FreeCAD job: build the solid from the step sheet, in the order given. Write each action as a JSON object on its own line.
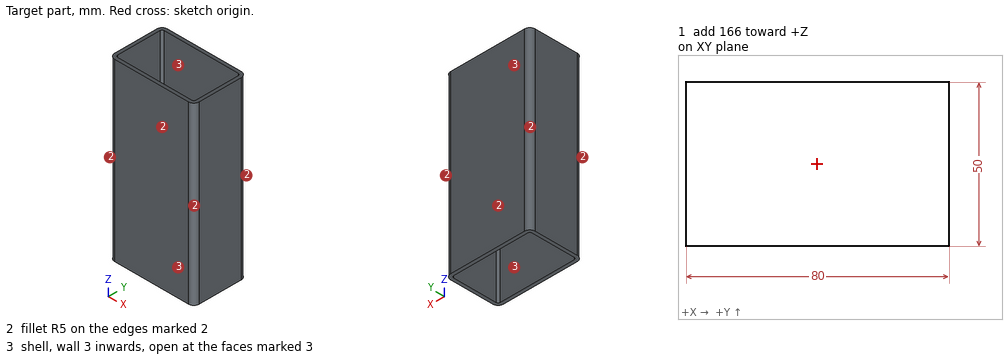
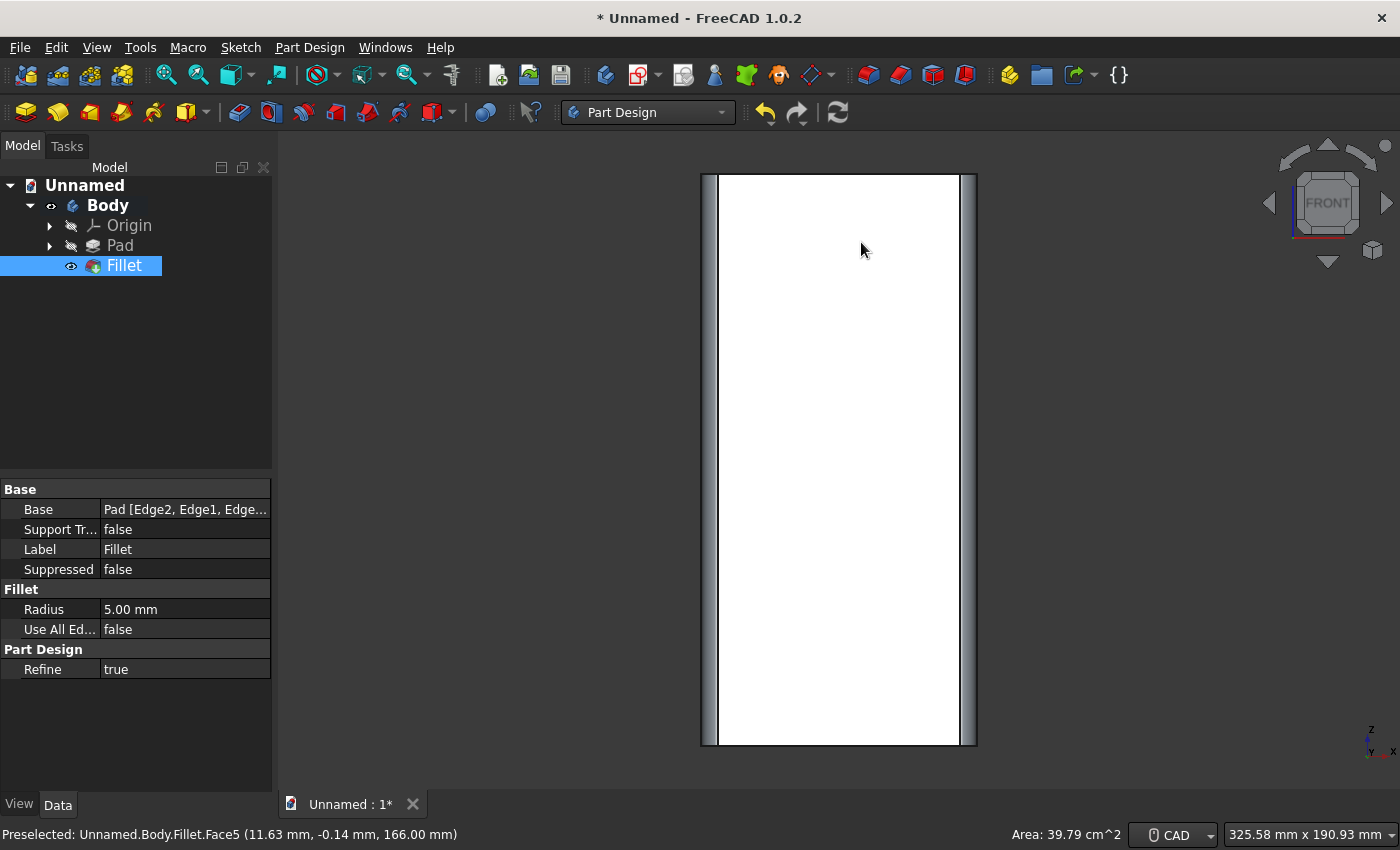
{"action": "key", "text": "3"}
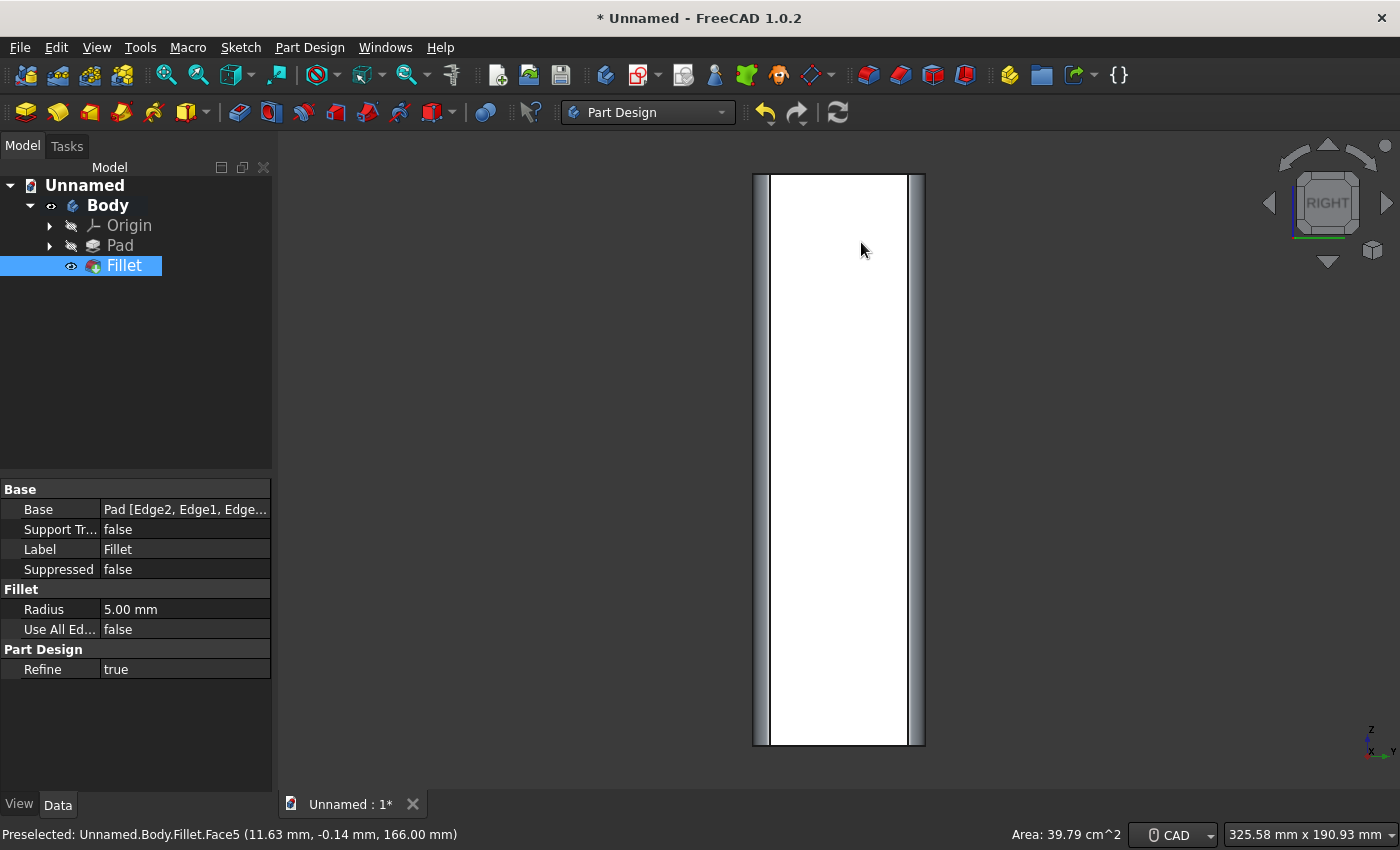
{"action": "key", "text": "5"}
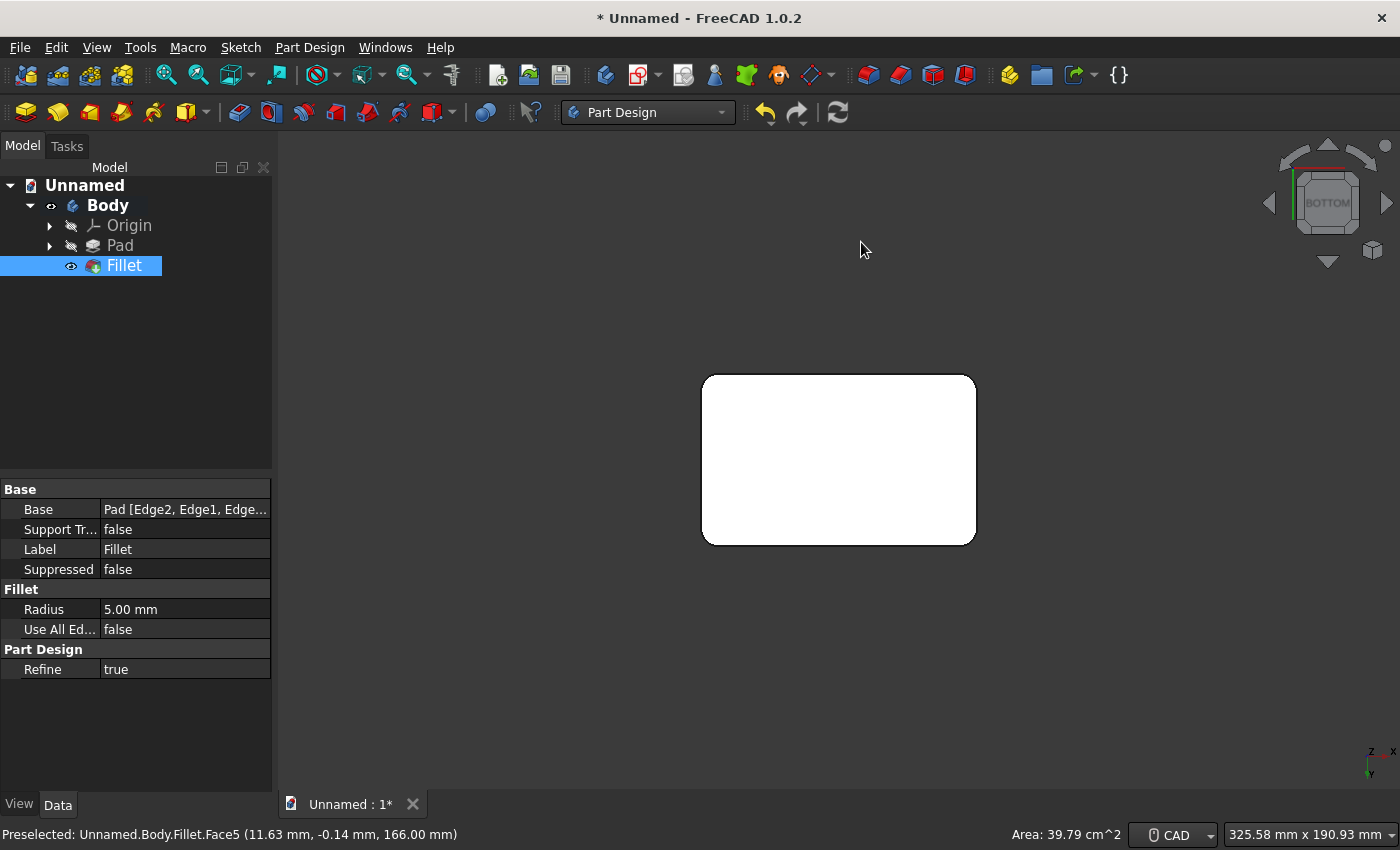
{"action": "left_click", "coordinate": [168, 76]}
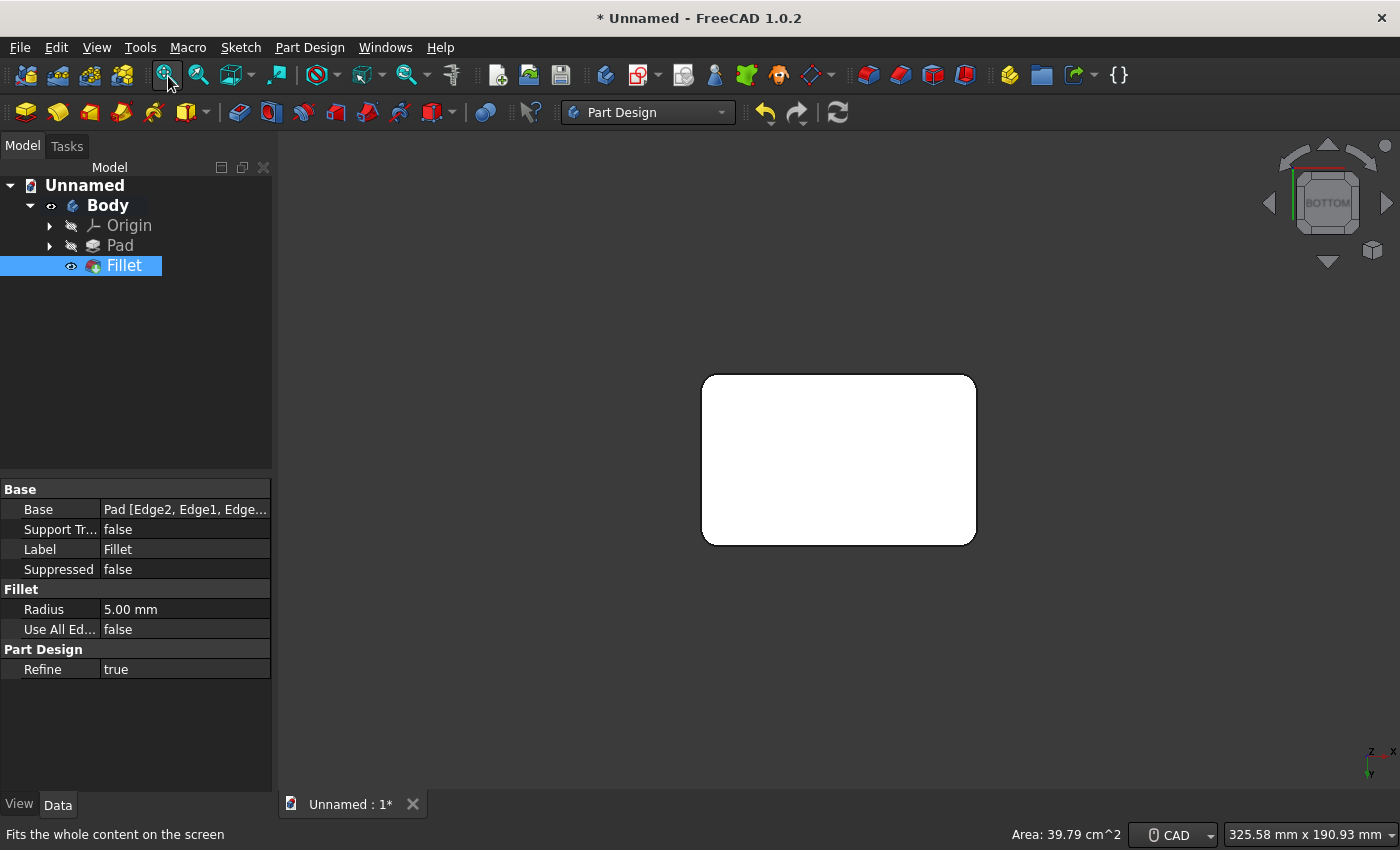
{"action": "left_click", "coordinate": [878, 459], "text": "ctrl"}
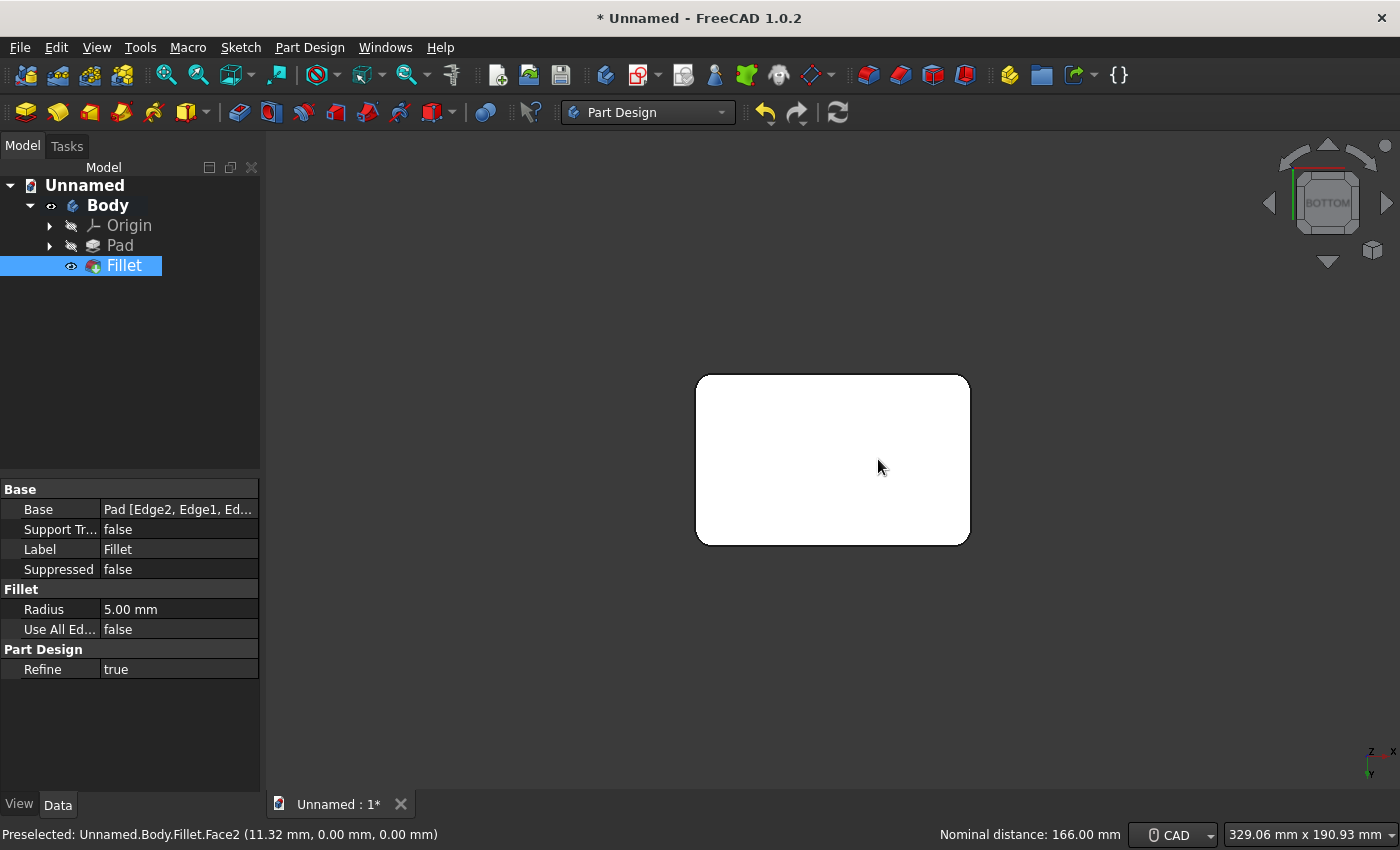
{"action": "left_click", "coordinate": [966, 76]}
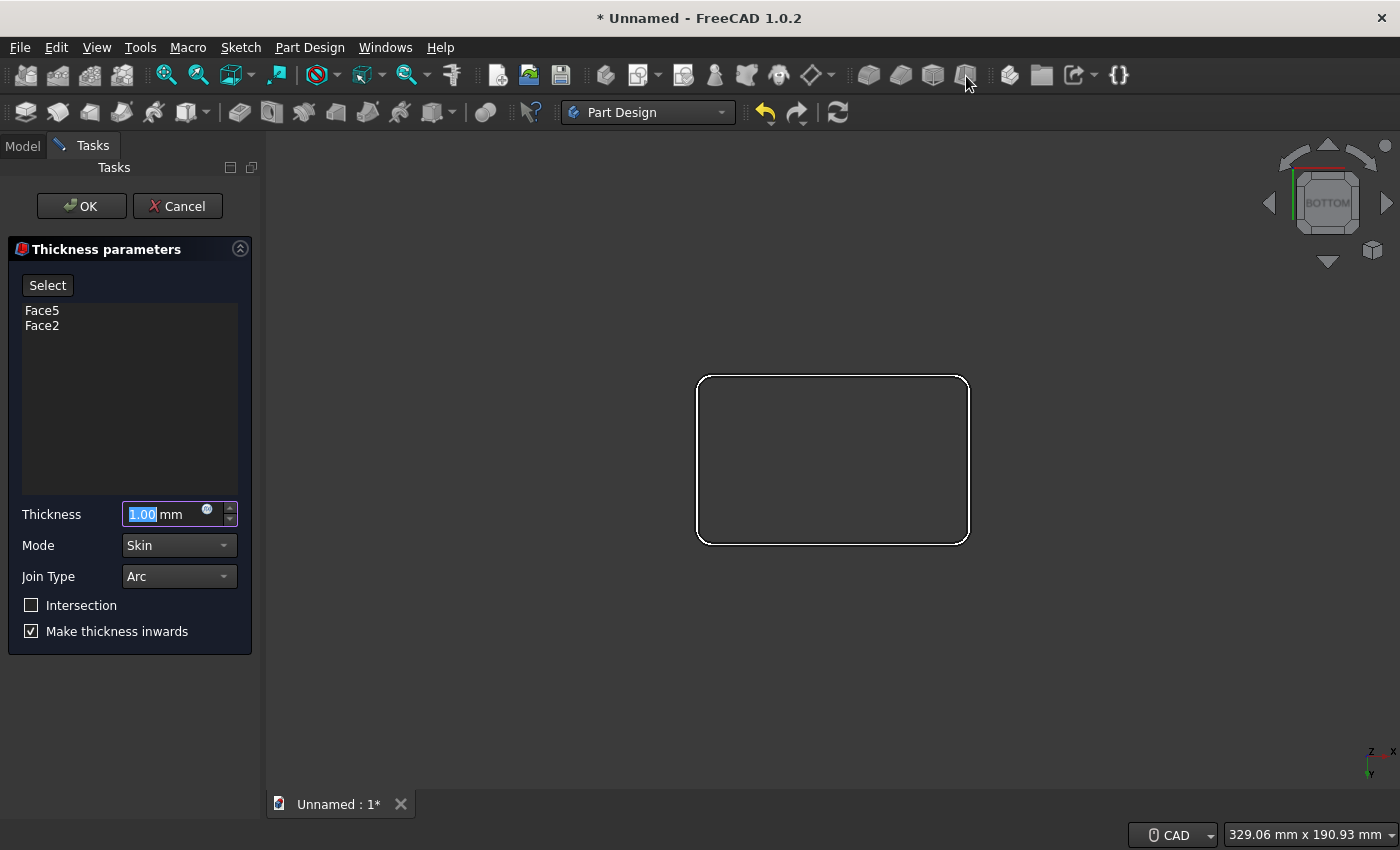
{"action": "type", "text": "3"}
{"action": "key", "text": "Tab"}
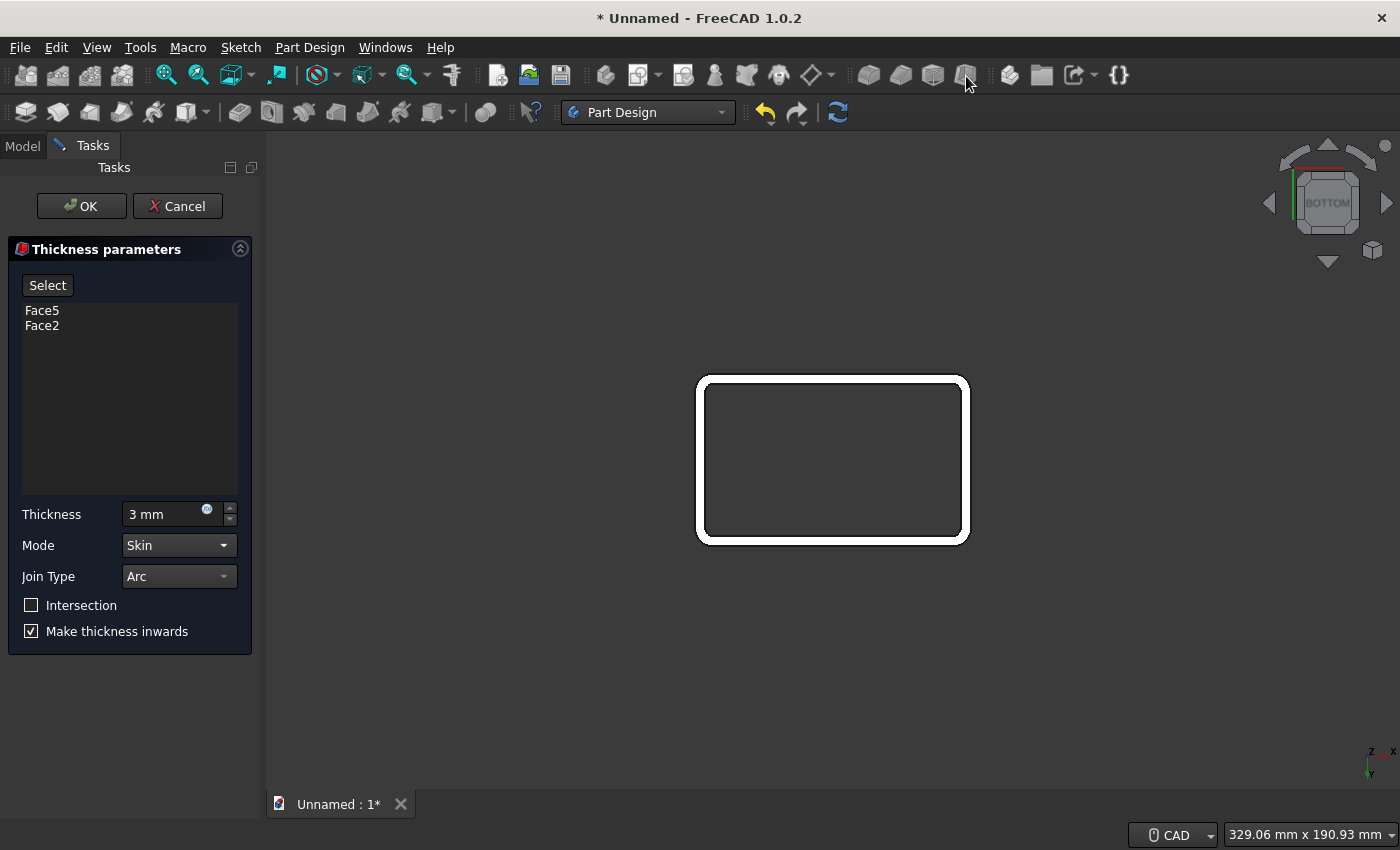
{"action": "left_click", "coordinate": [180, 576]}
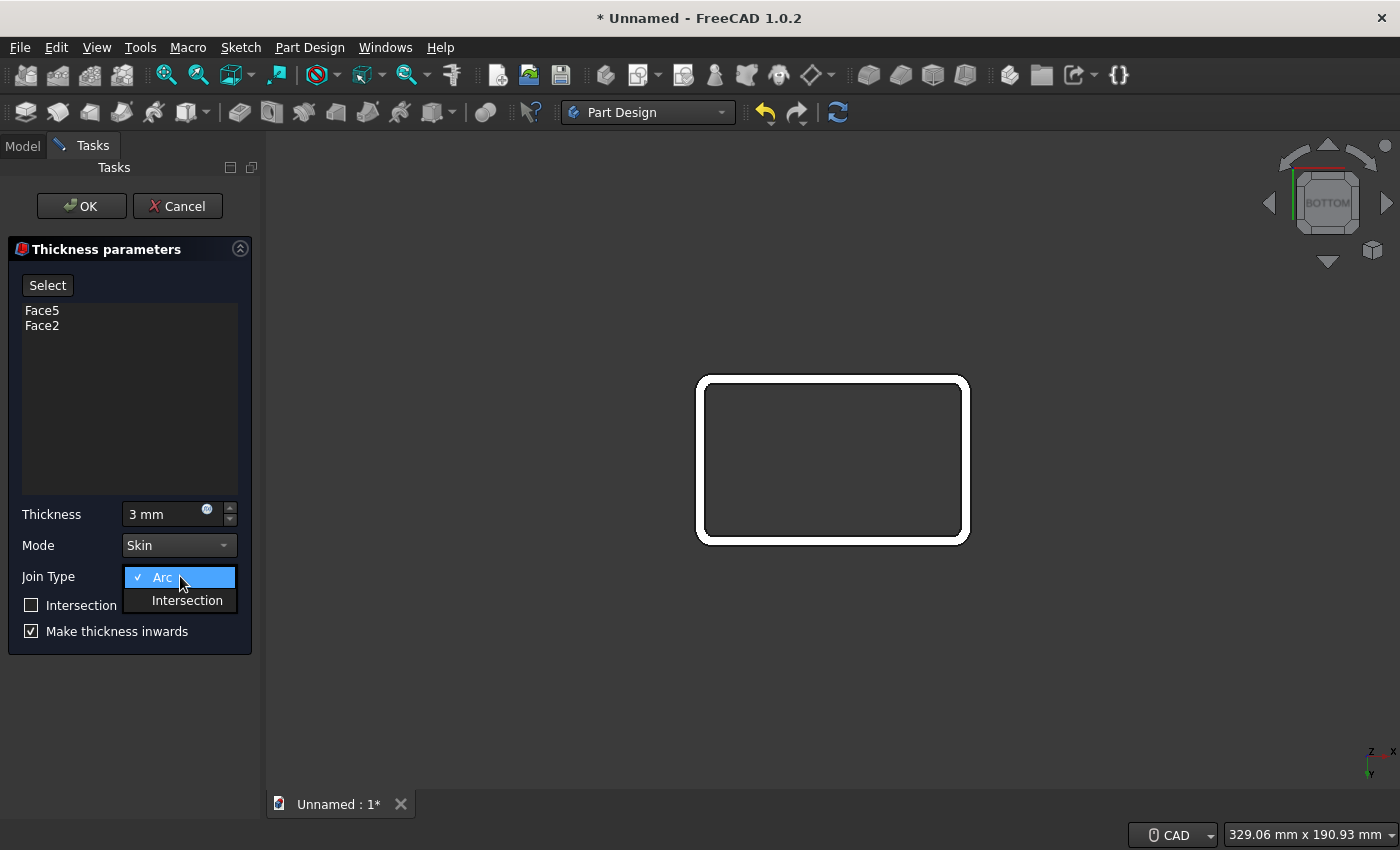
{"action": "left_click", "coordinate": [179, 600]}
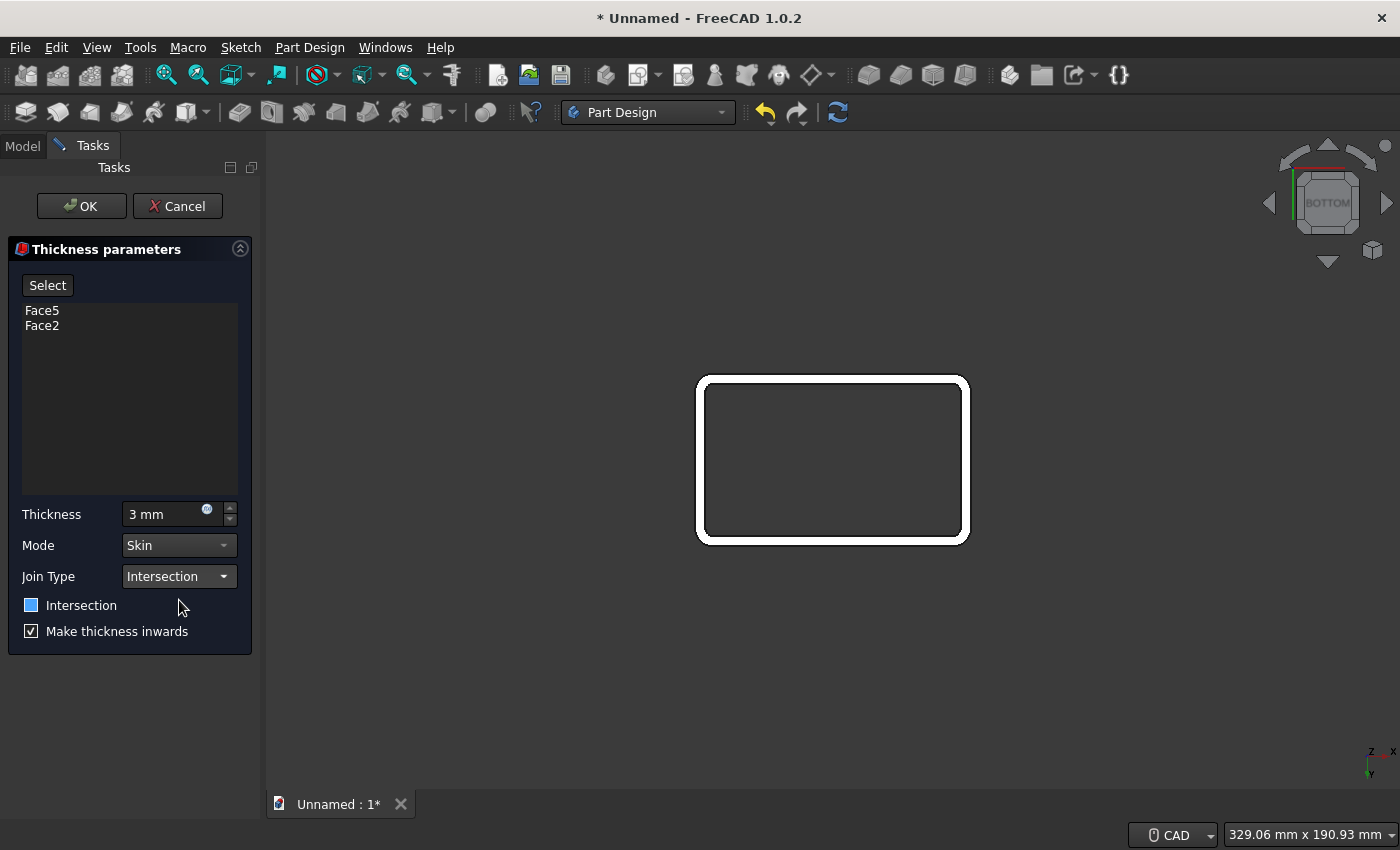
{"action": "left_click", "coordinate": [82, 206]}